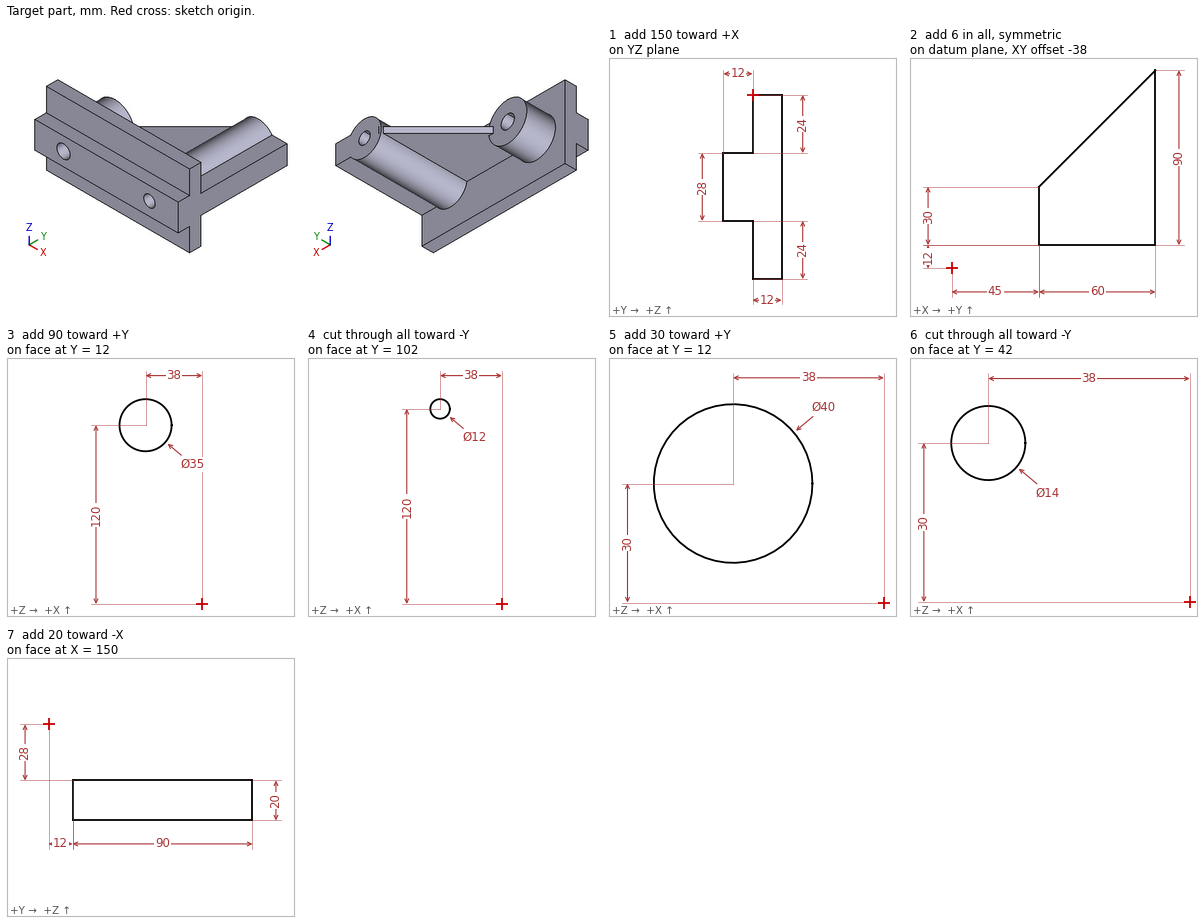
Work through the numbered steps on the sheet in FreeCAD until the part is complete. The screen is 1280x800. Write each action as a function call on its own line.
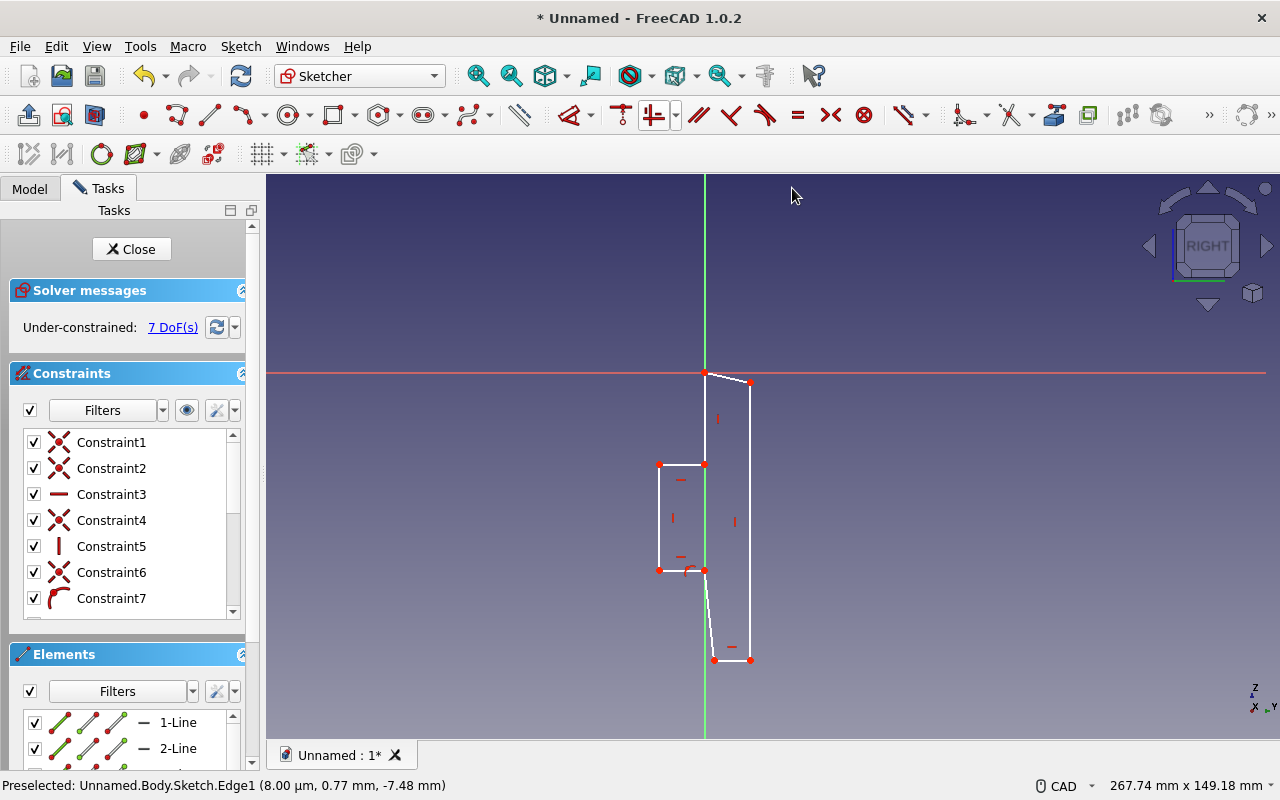
click(707, 598)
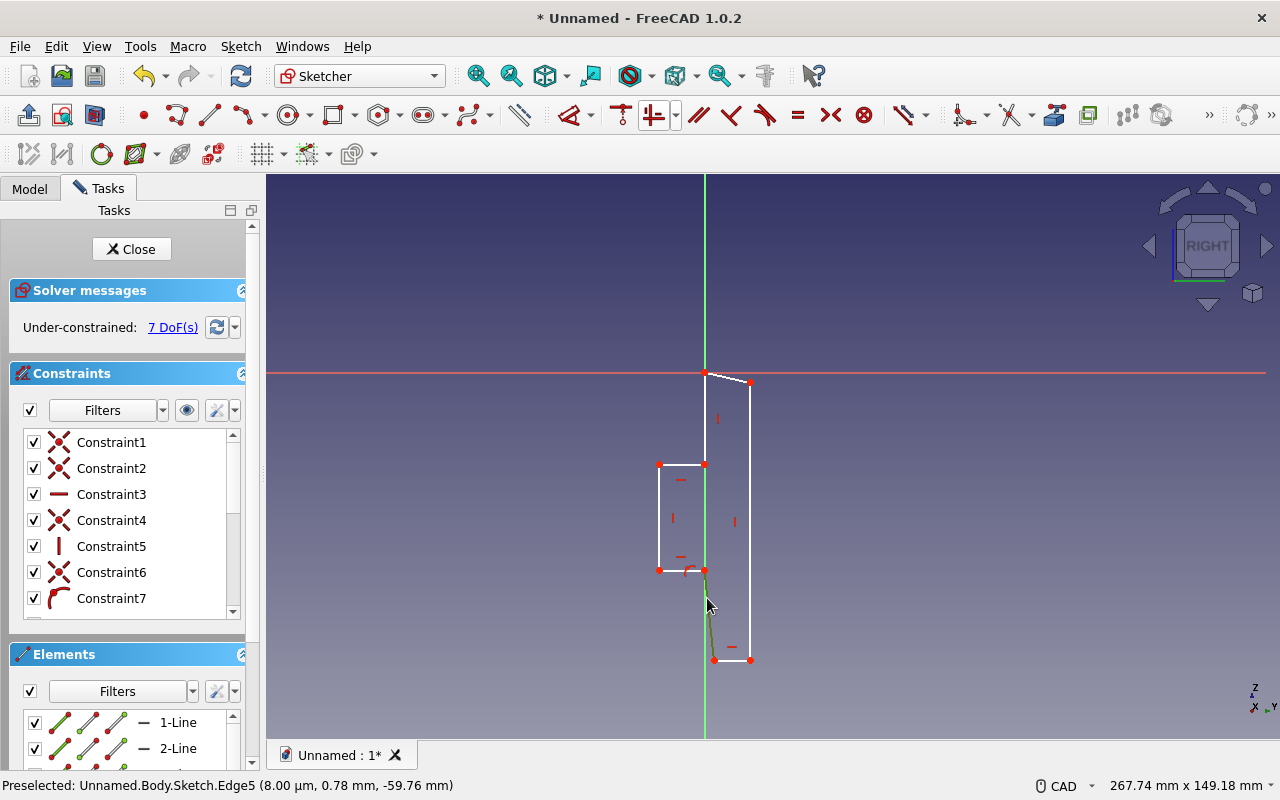
click(676, 116)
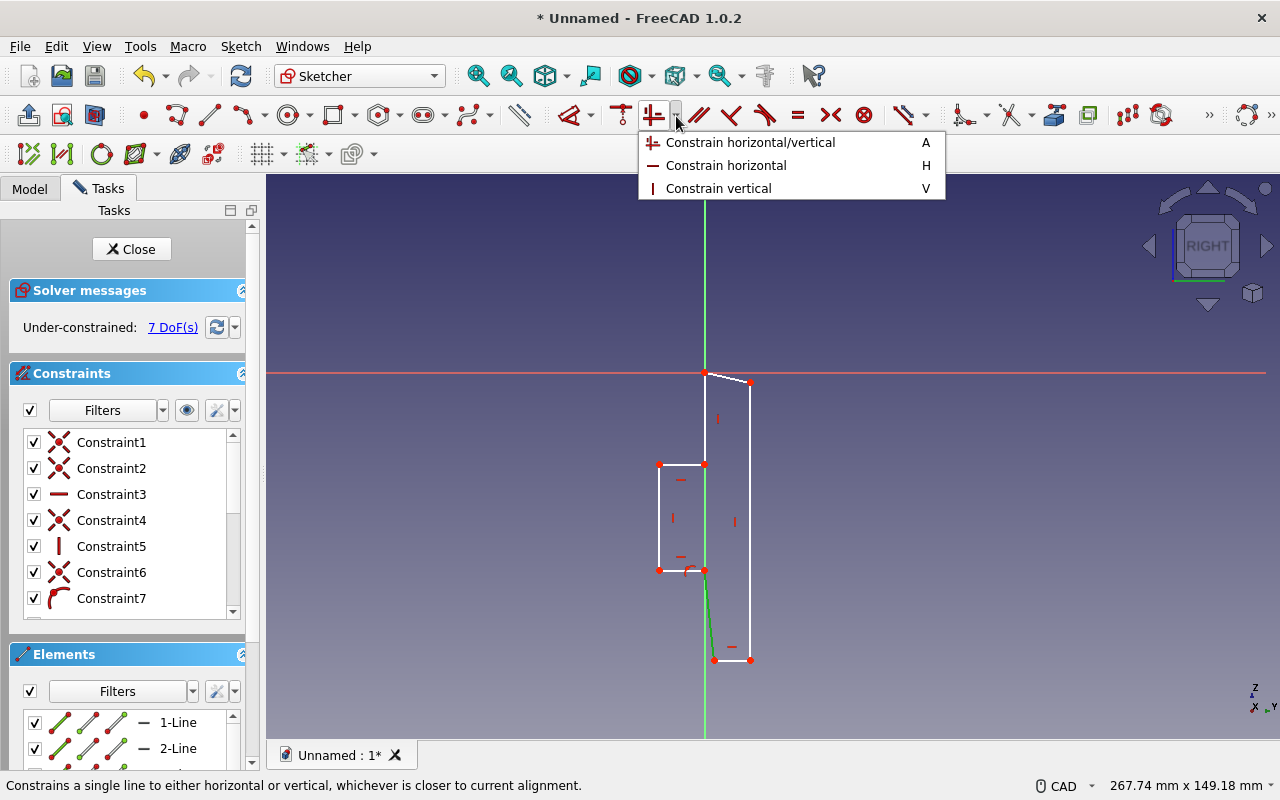
click(792, 188)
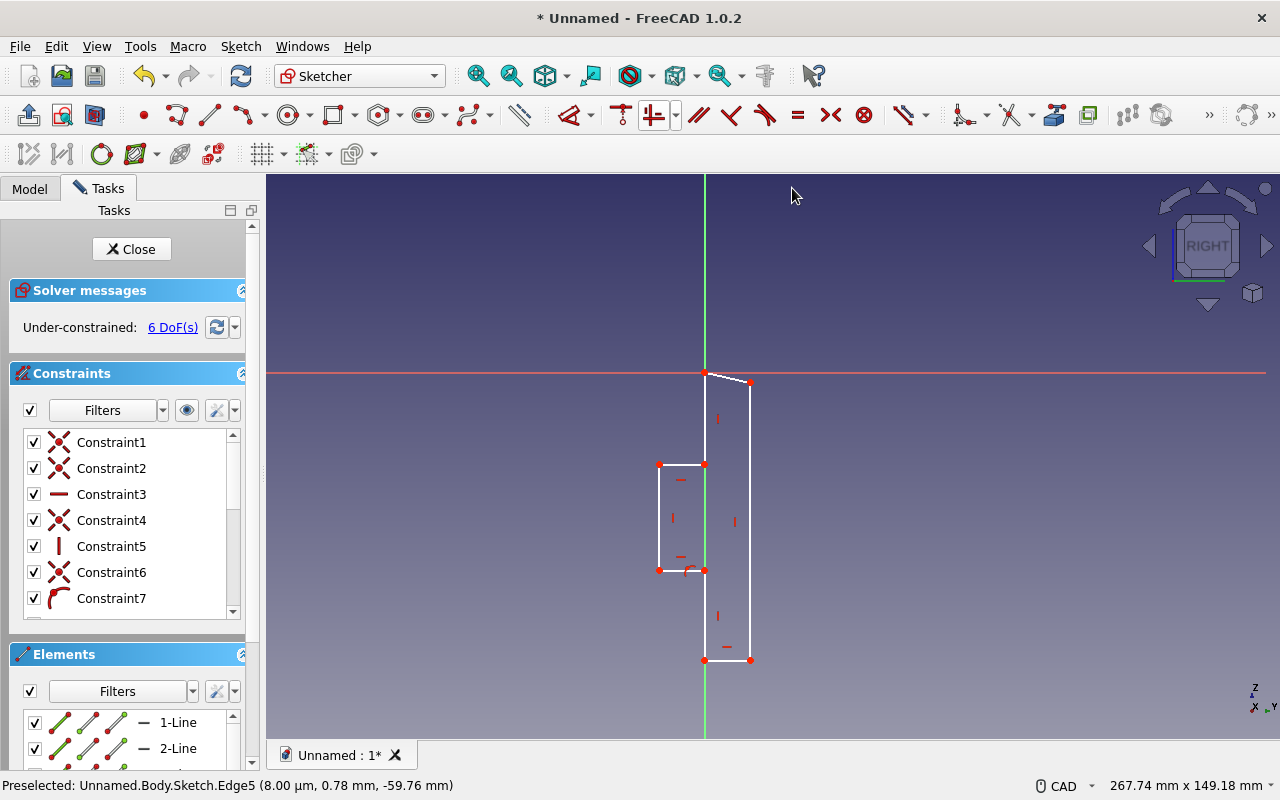
click(718, 376)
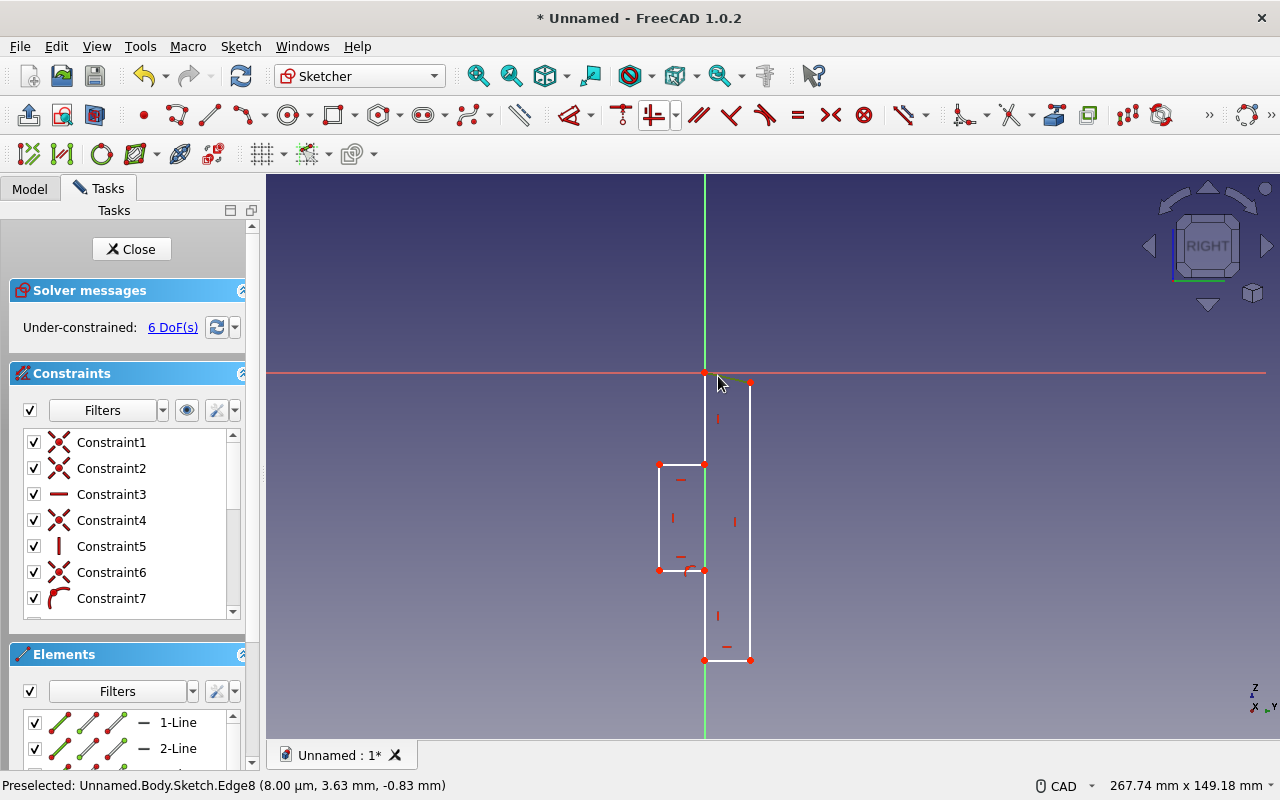
key(h)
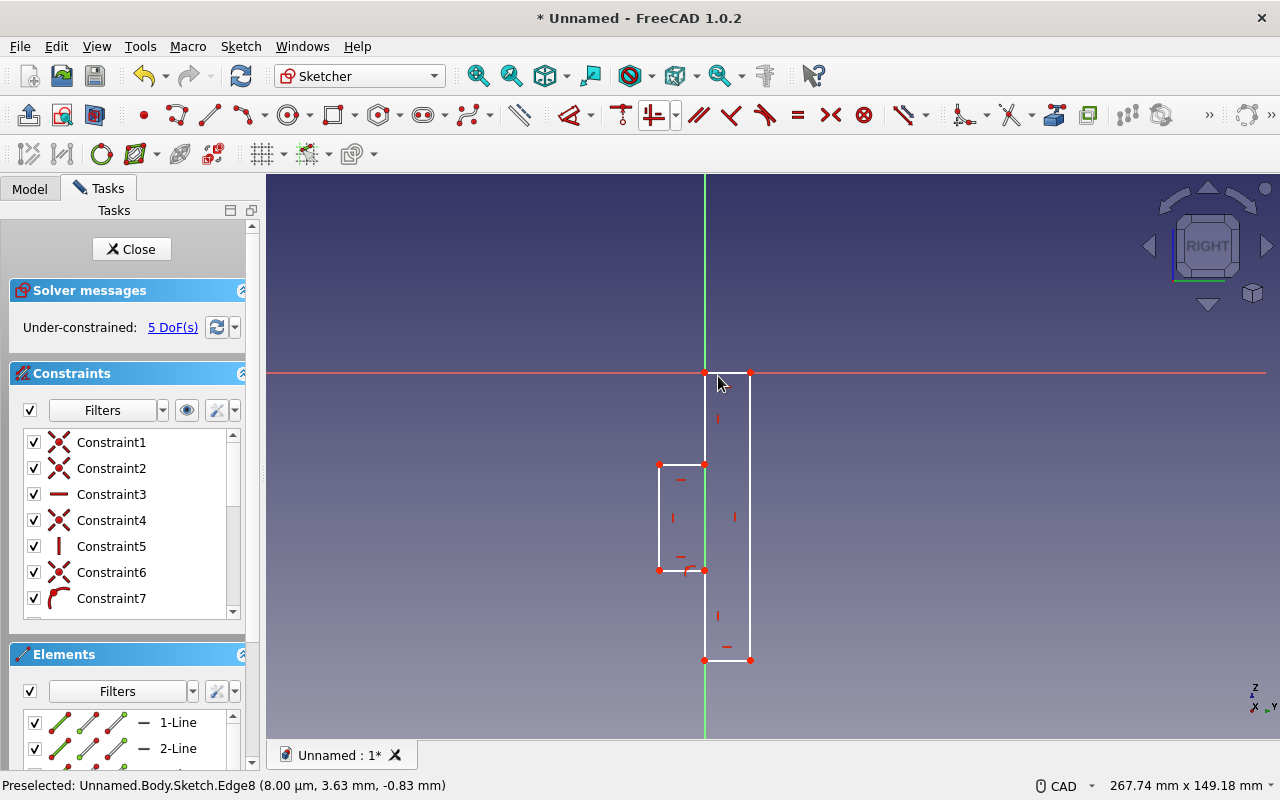
click(568, 116)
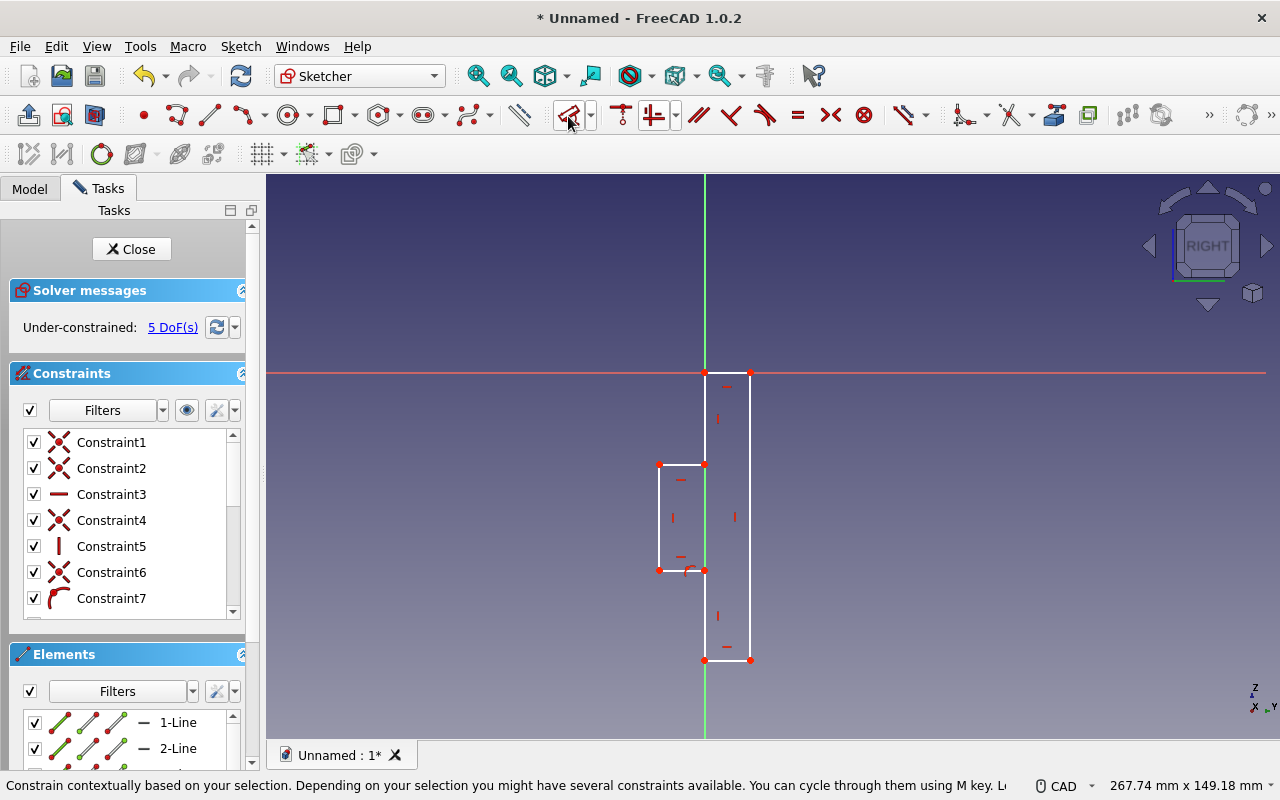
click(705, 400)
click(671, 419)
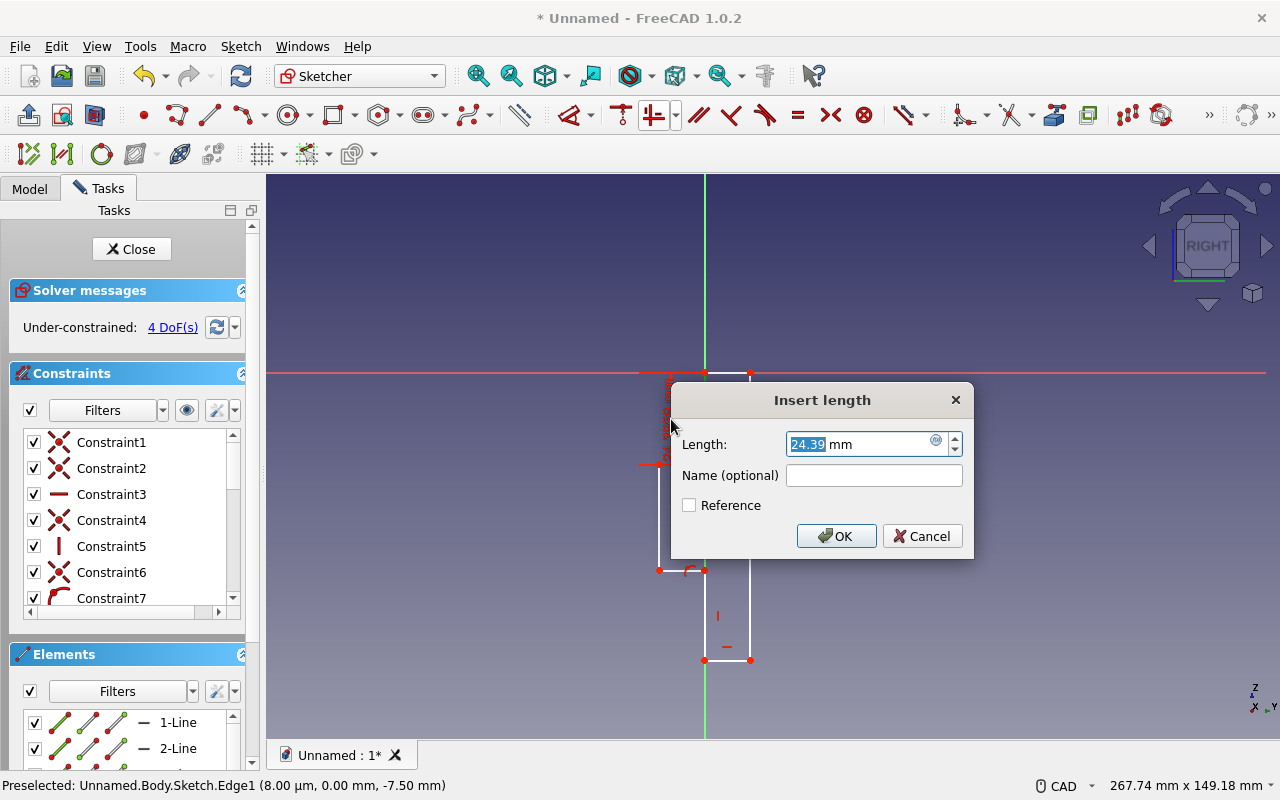
text(24)
key(Return)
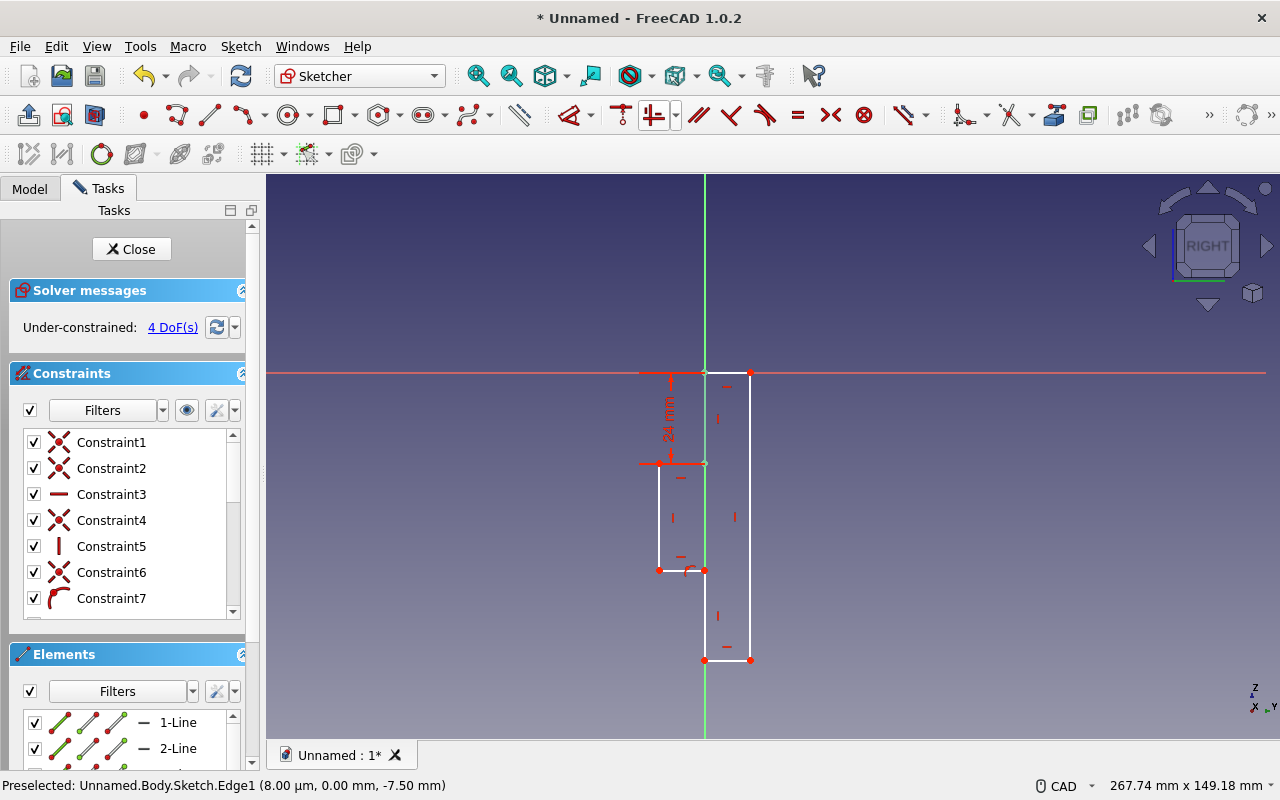
click(691, 464)
click(682, 498)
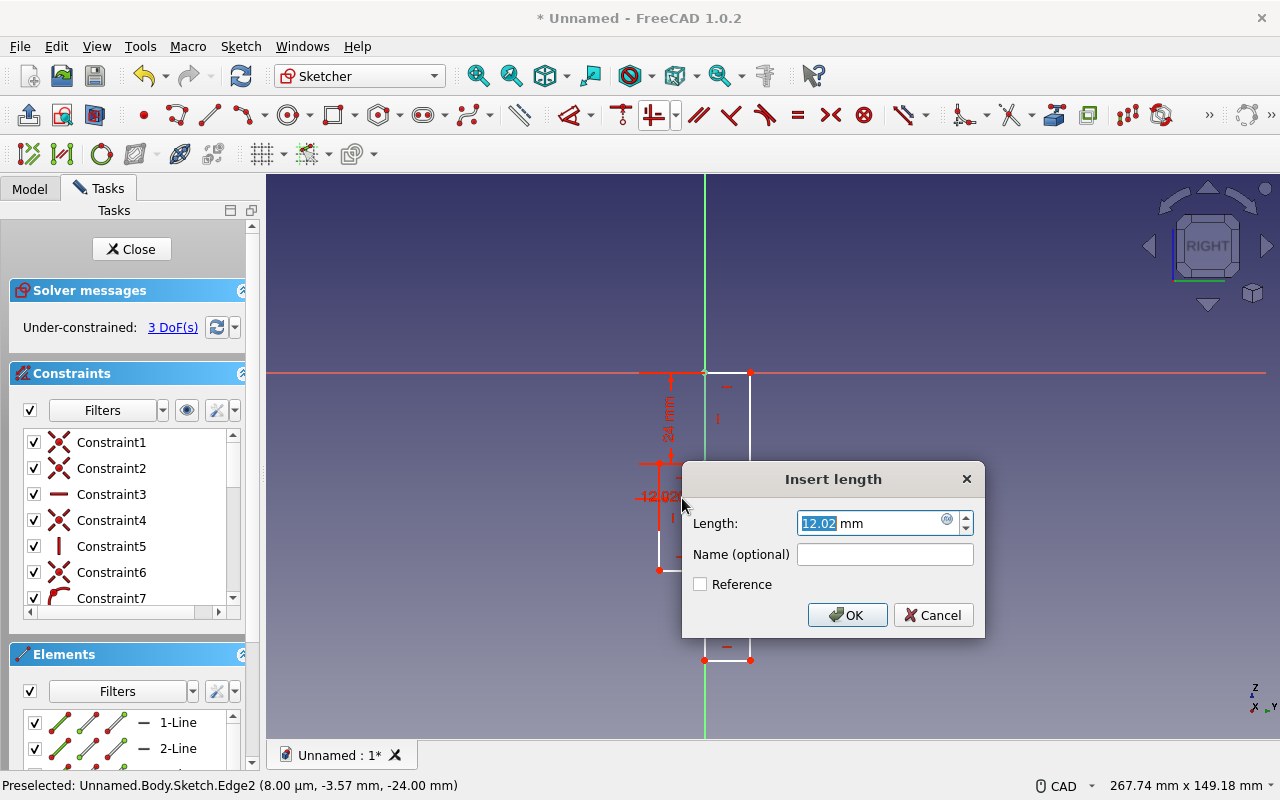
text(12)
key(Return)